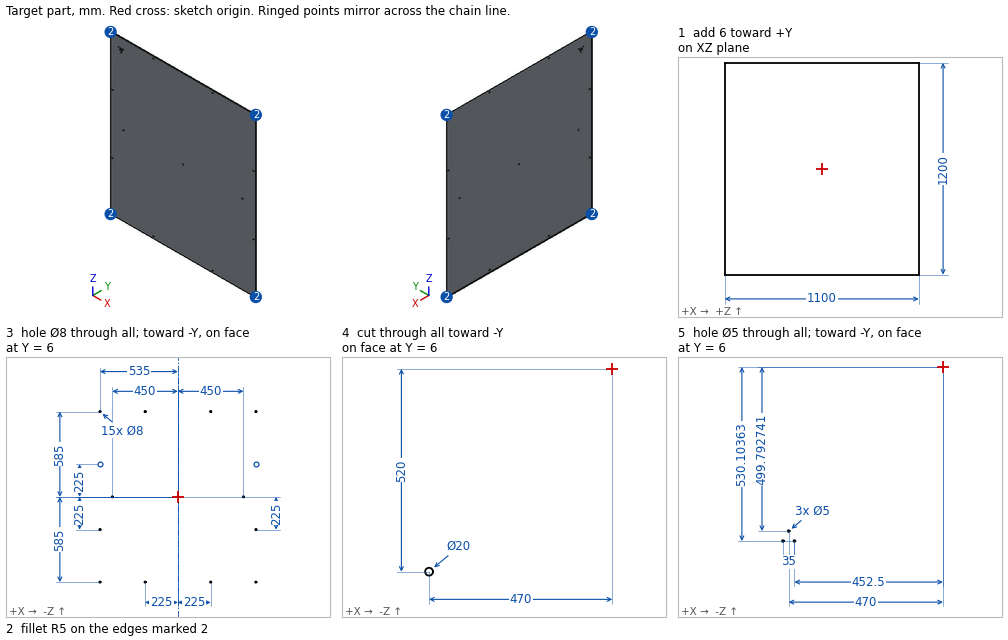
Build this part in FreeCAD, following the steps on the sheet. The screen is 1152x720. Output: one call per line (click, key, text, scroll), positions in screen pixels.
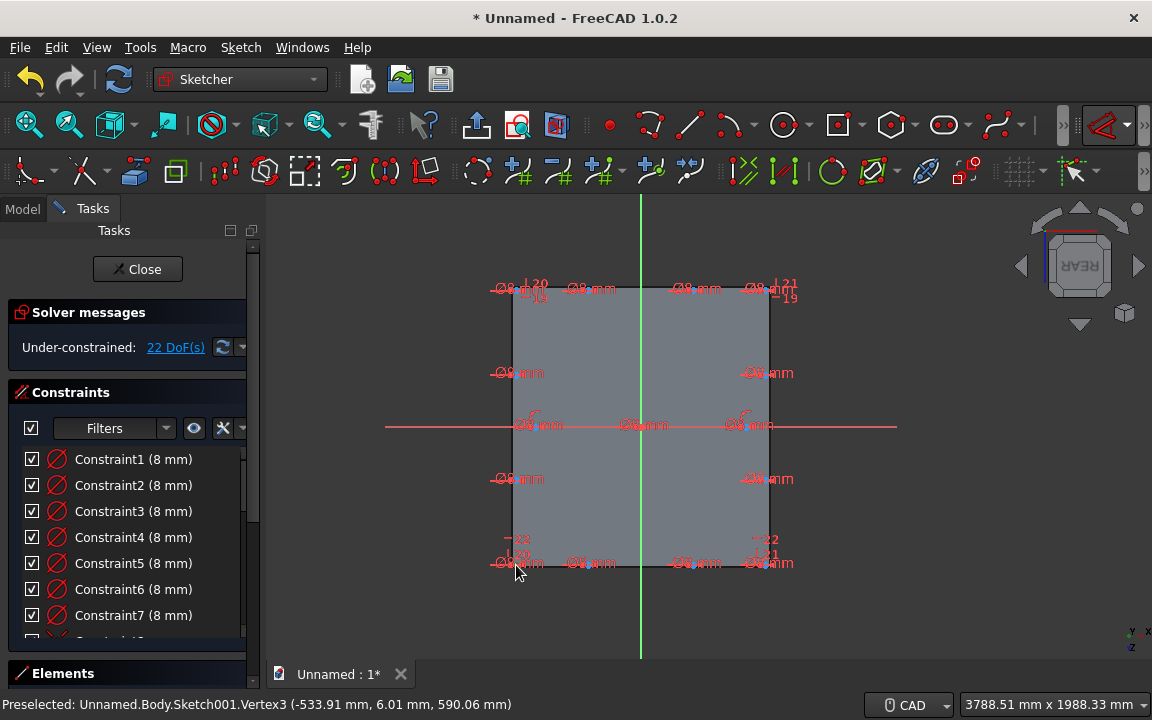
click(588, 565)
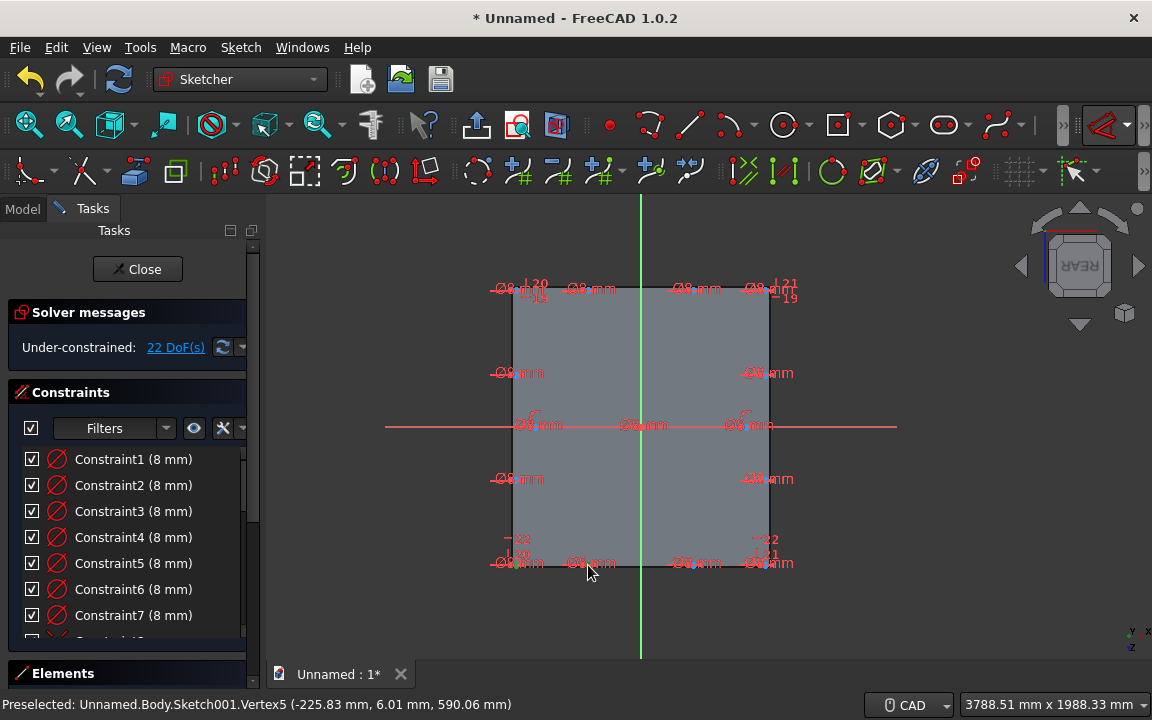
key(h)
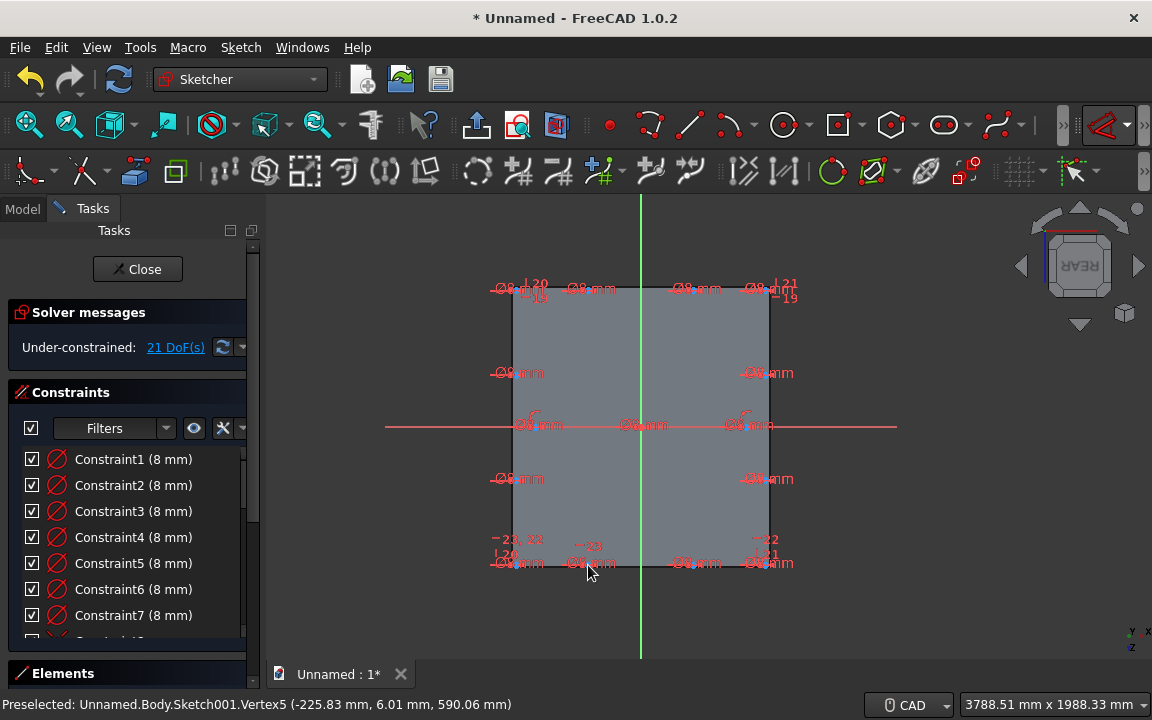
click(766, 565)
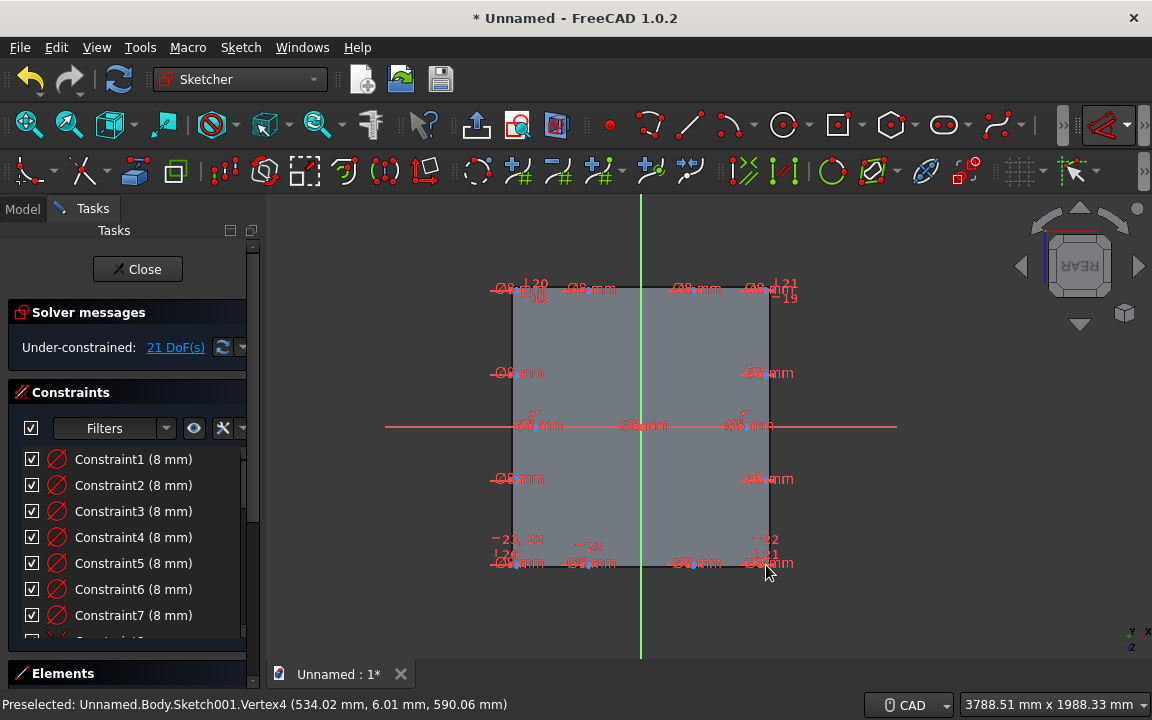
click(694, 565)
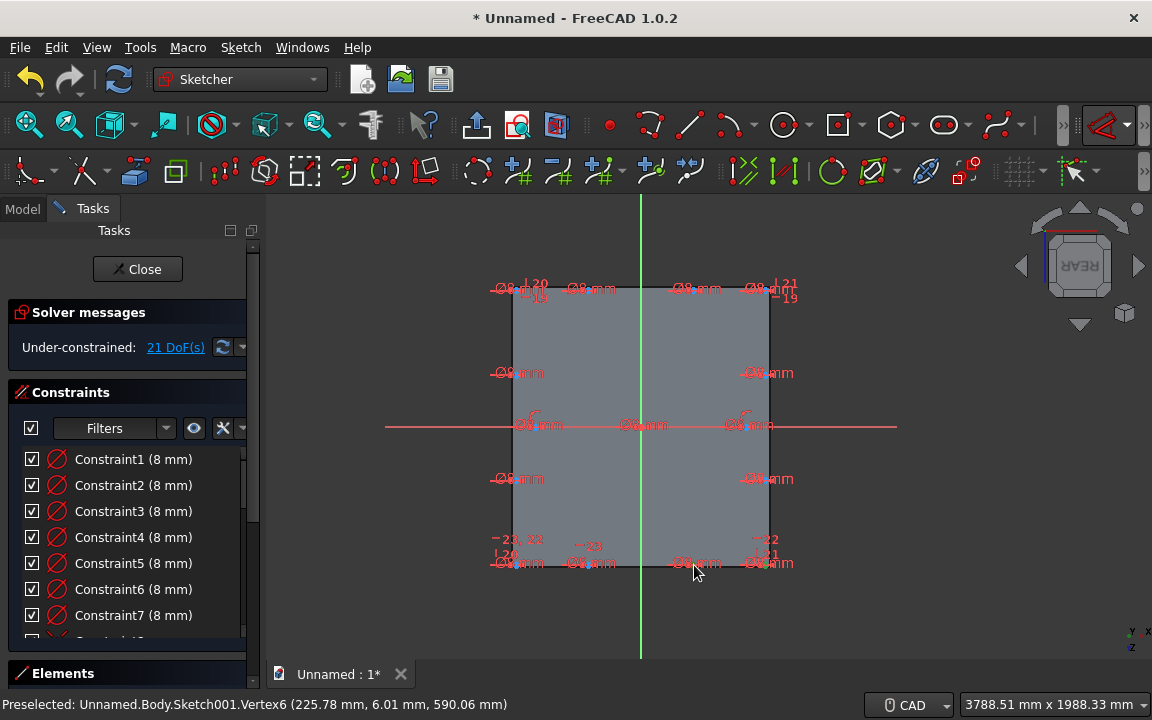
key(h)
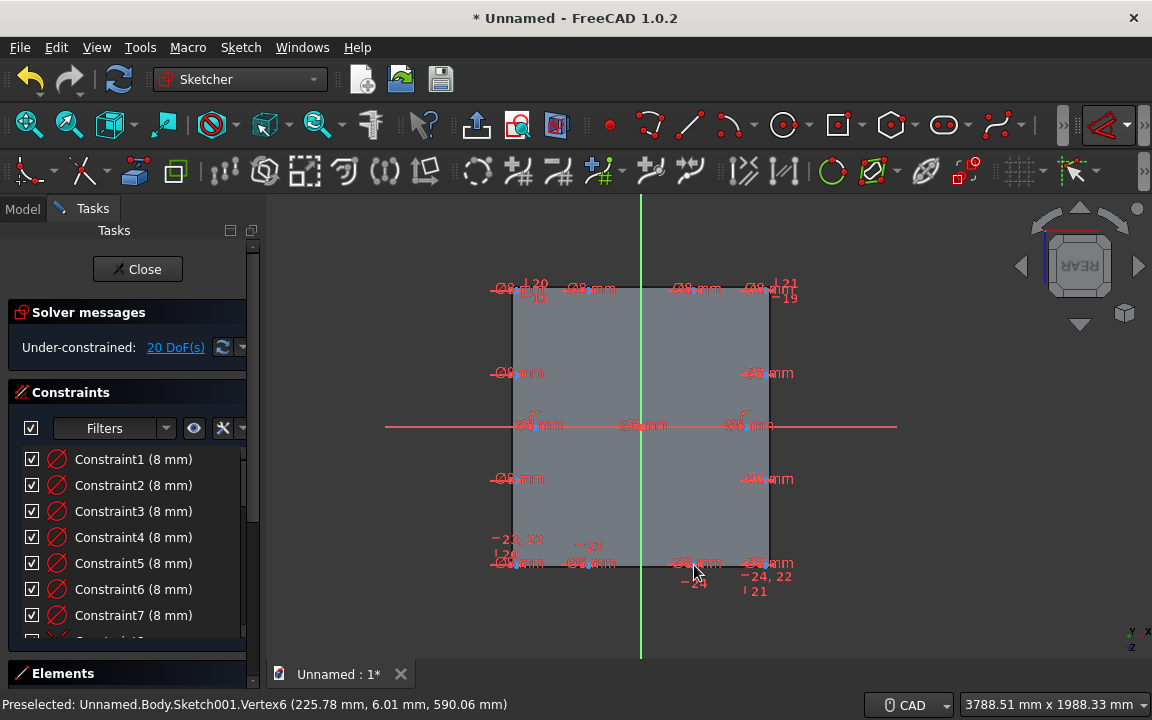
click(588, 565)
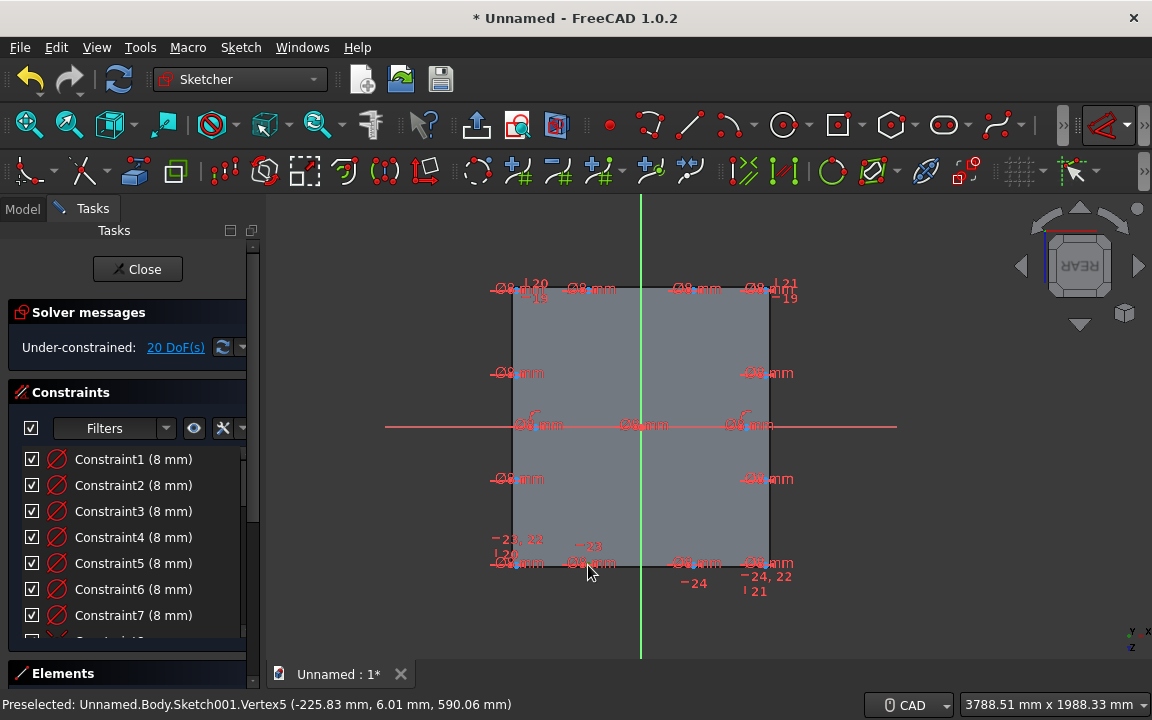
click(588, 291)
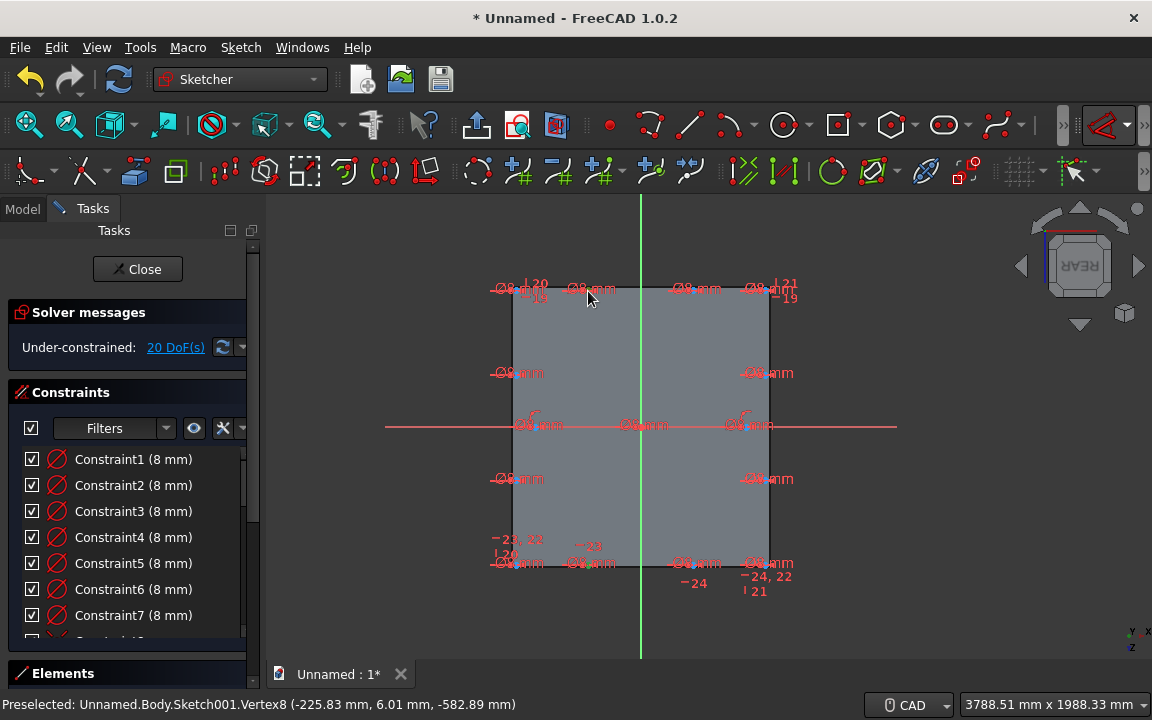
key(v)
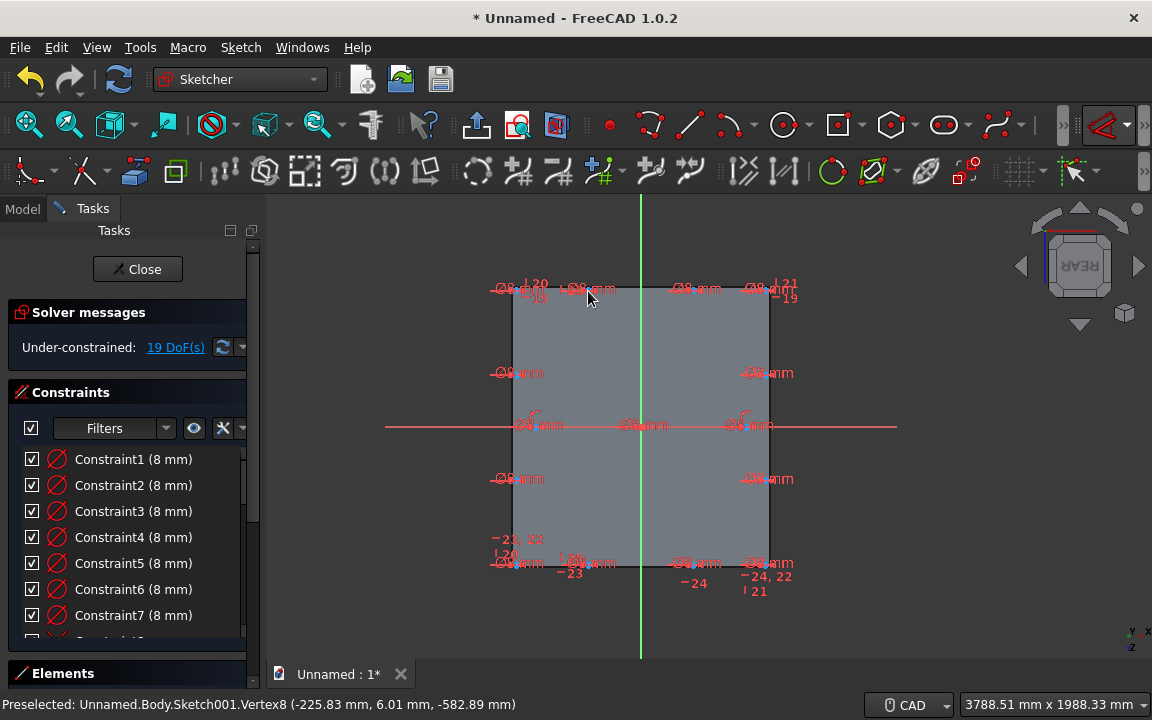
click(516, 291)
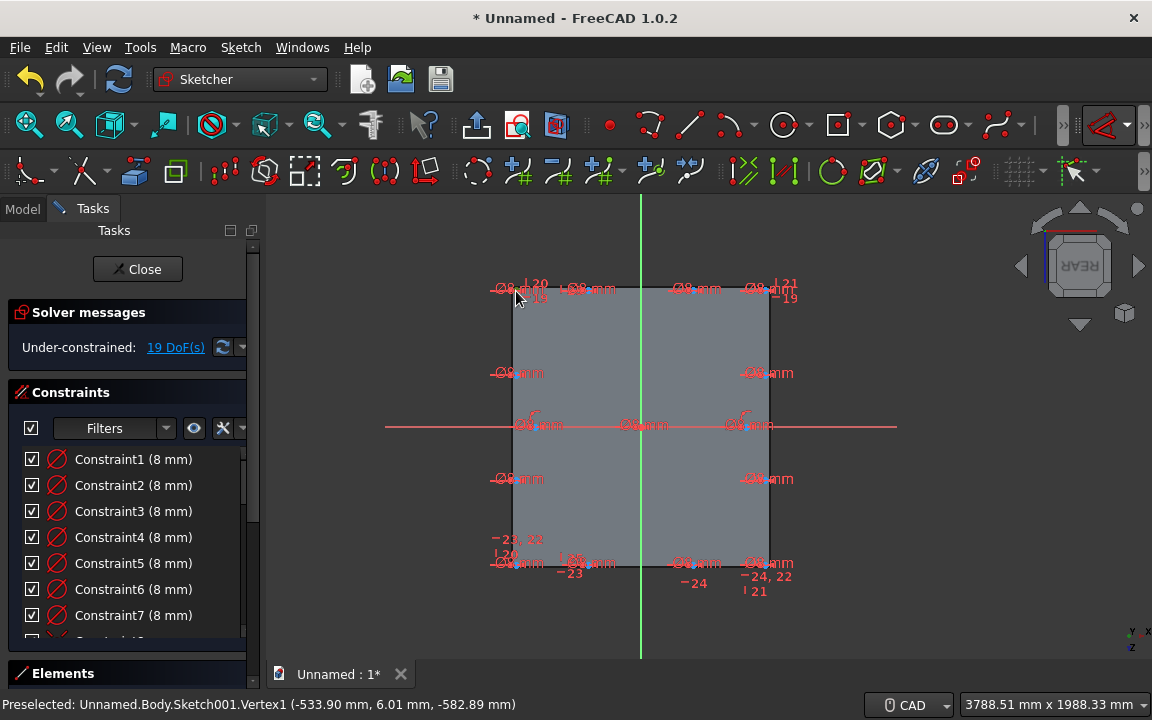
click(588, 291)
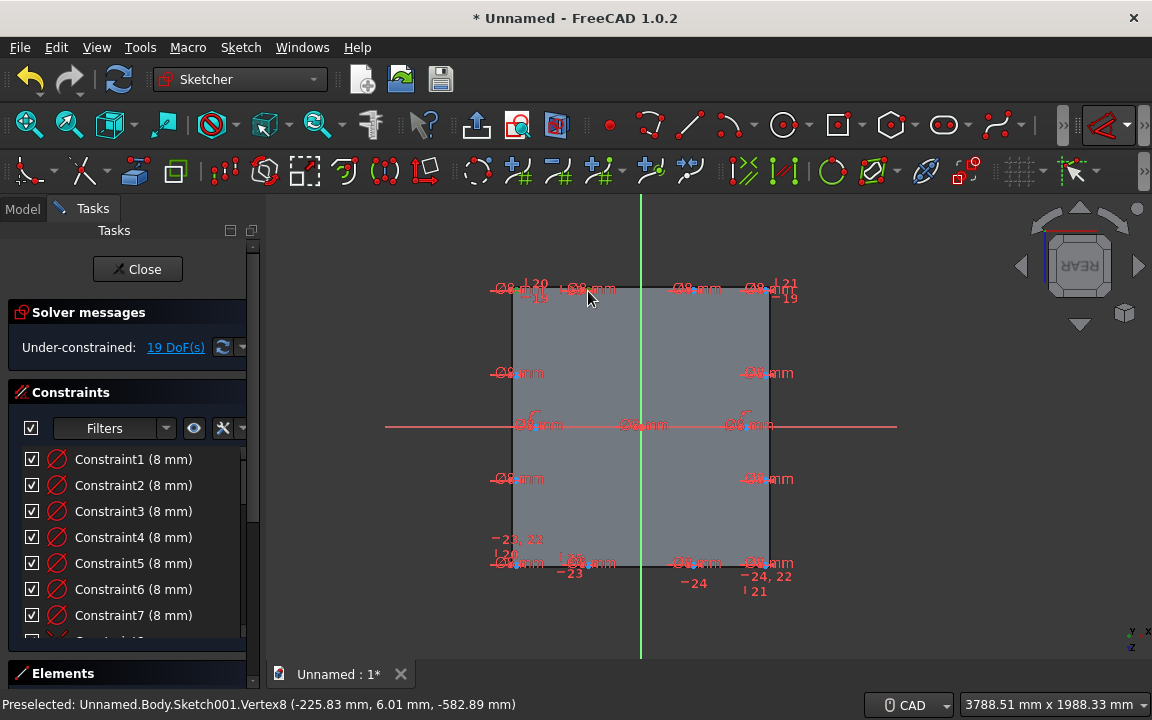
key(h)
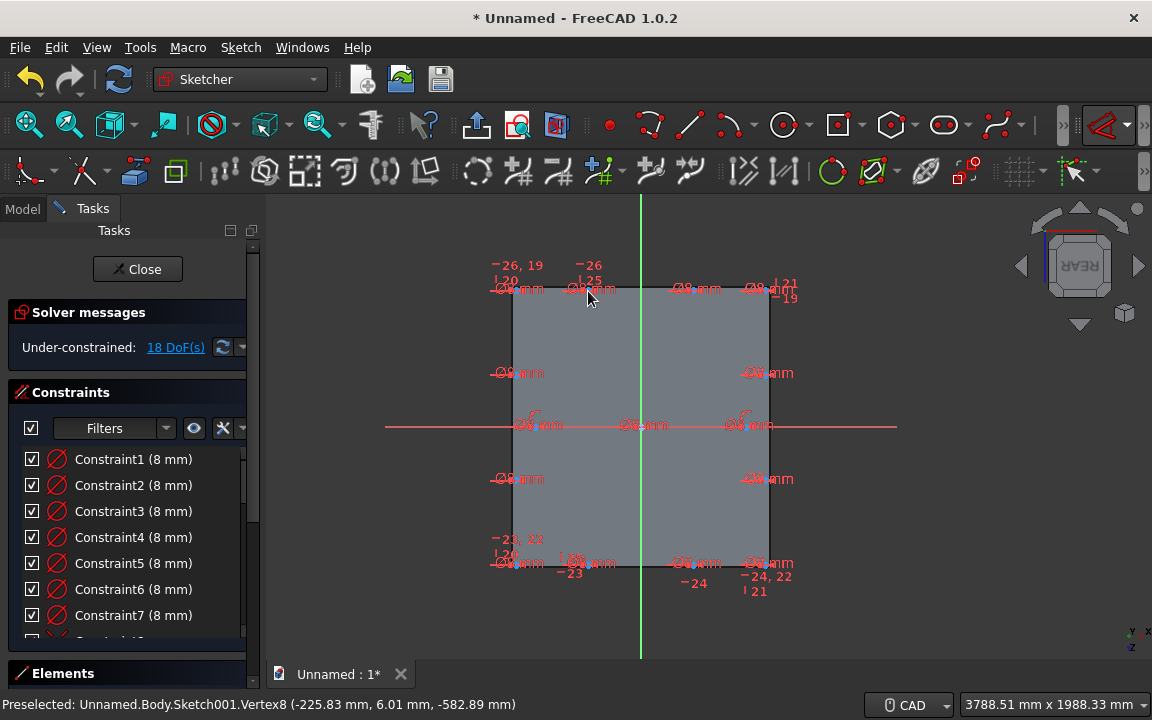
click(694, 565)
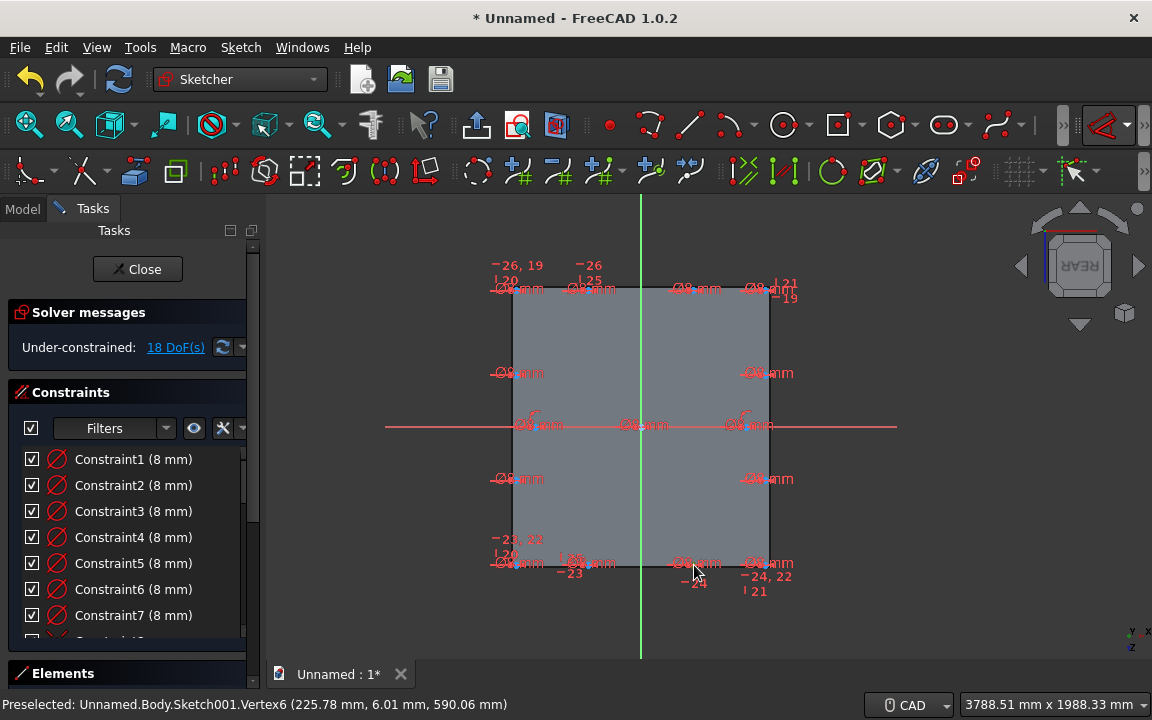
click(694, 291)